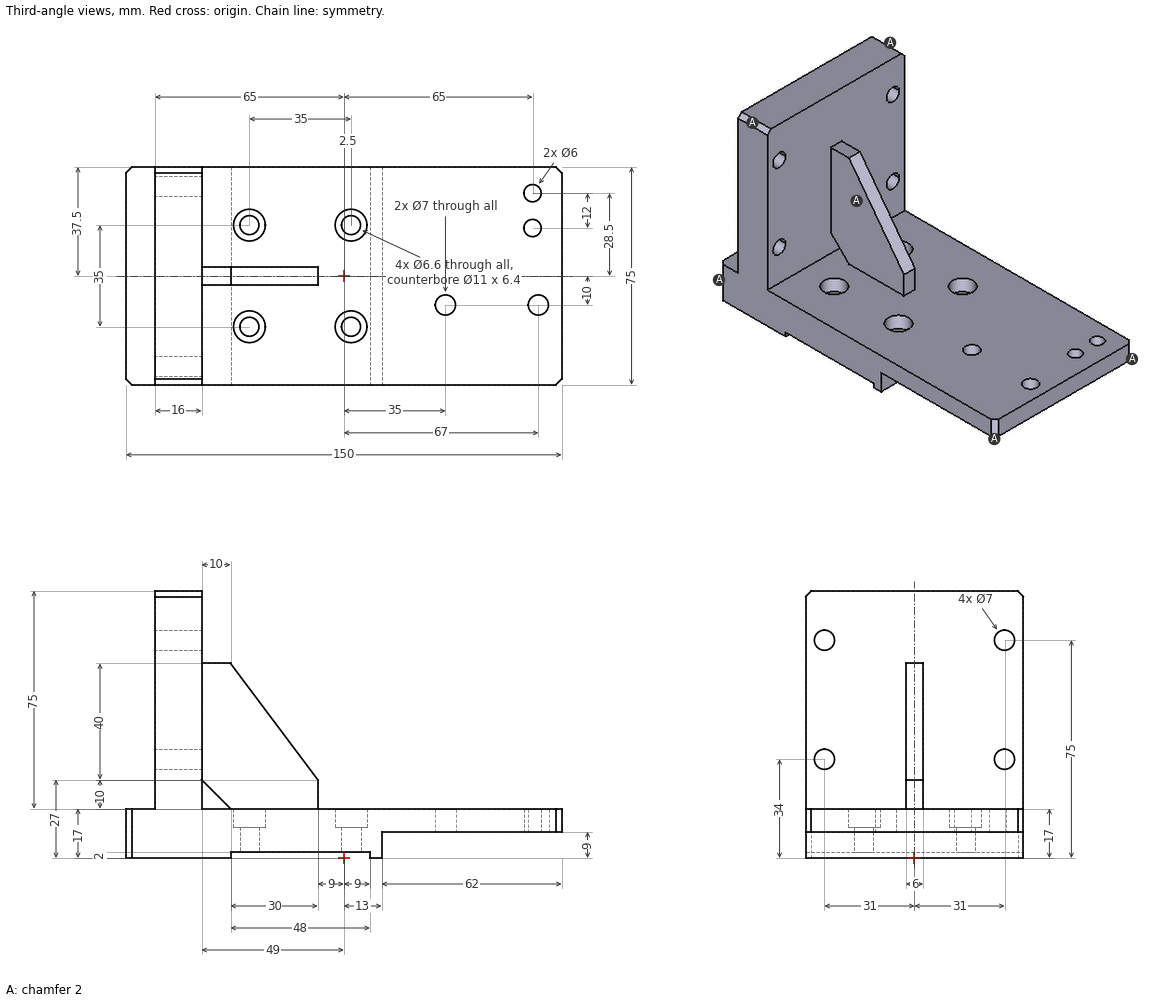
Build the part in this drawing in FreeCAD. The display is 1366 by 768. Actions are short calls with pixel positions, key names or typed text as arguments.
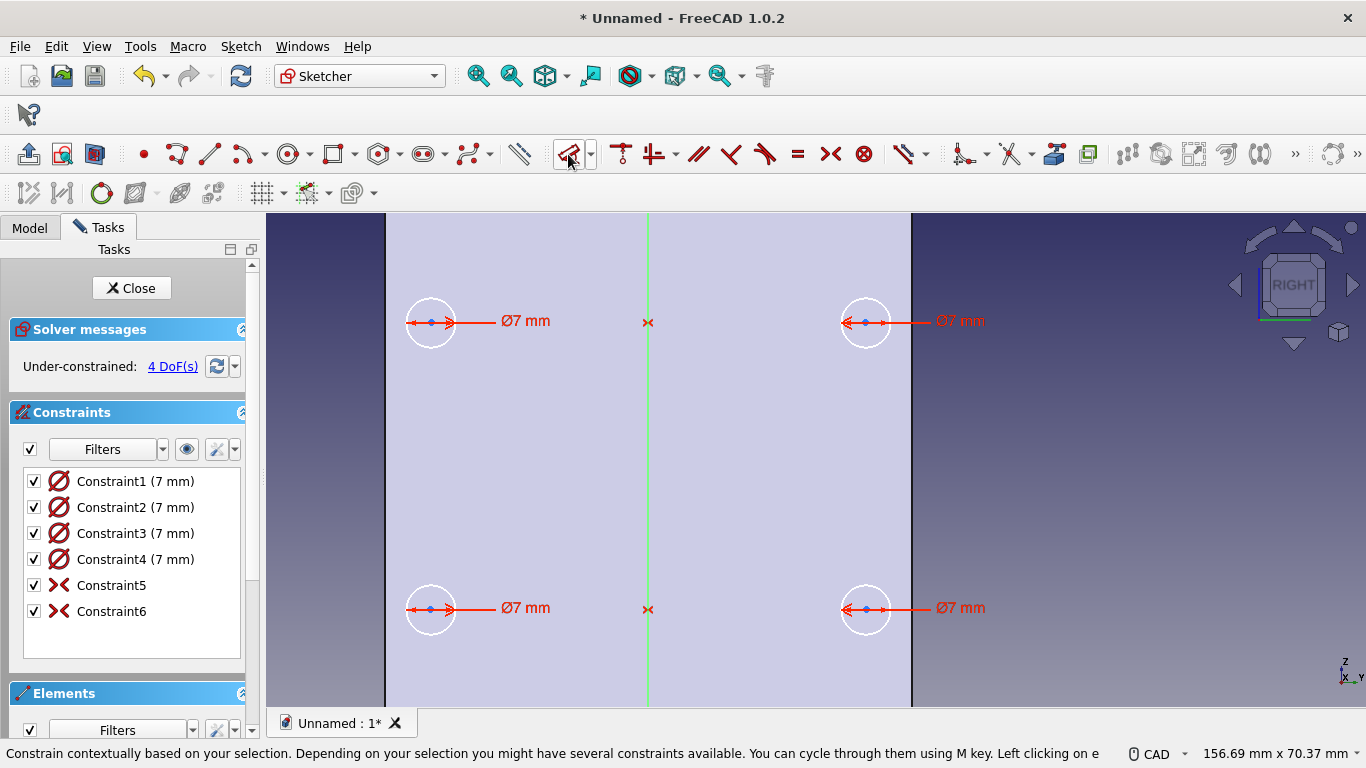
click(866, 323)
click(757, 289)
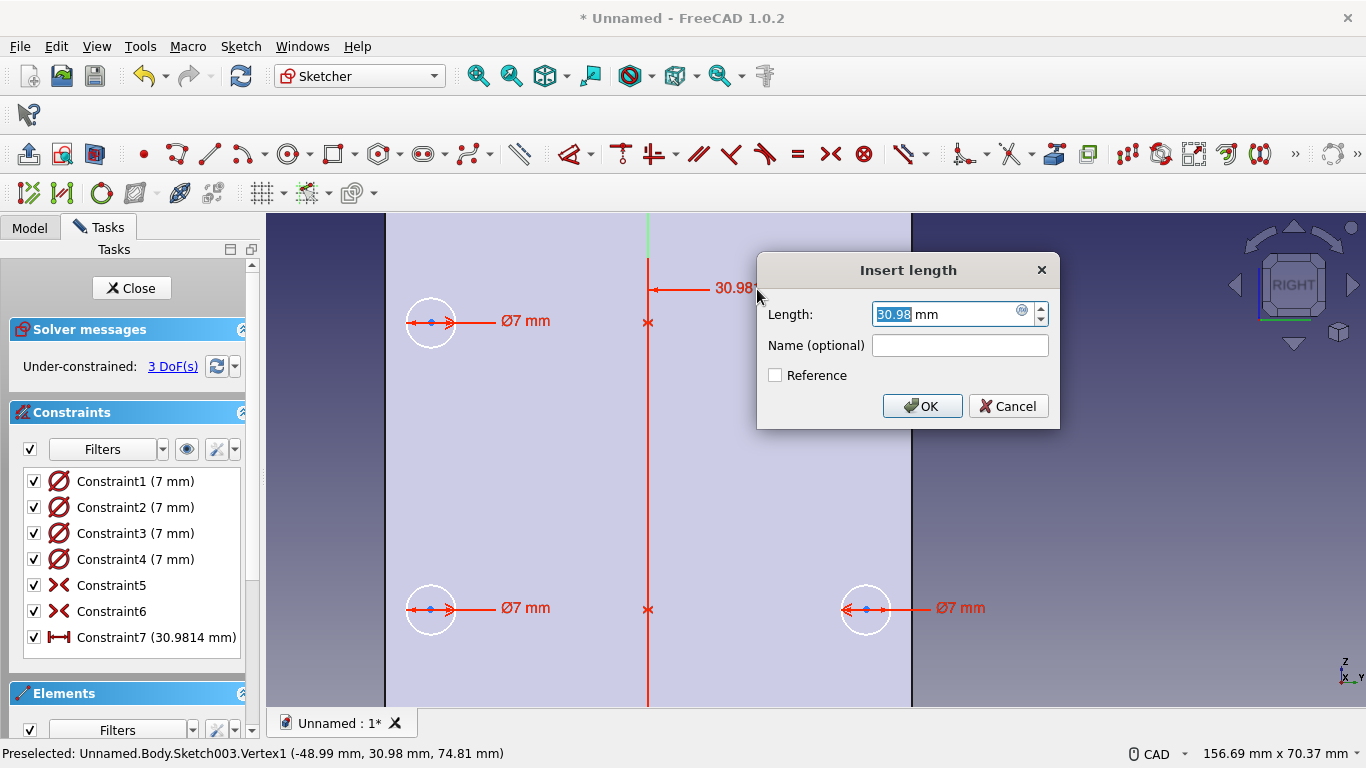
text(31)
key(Return)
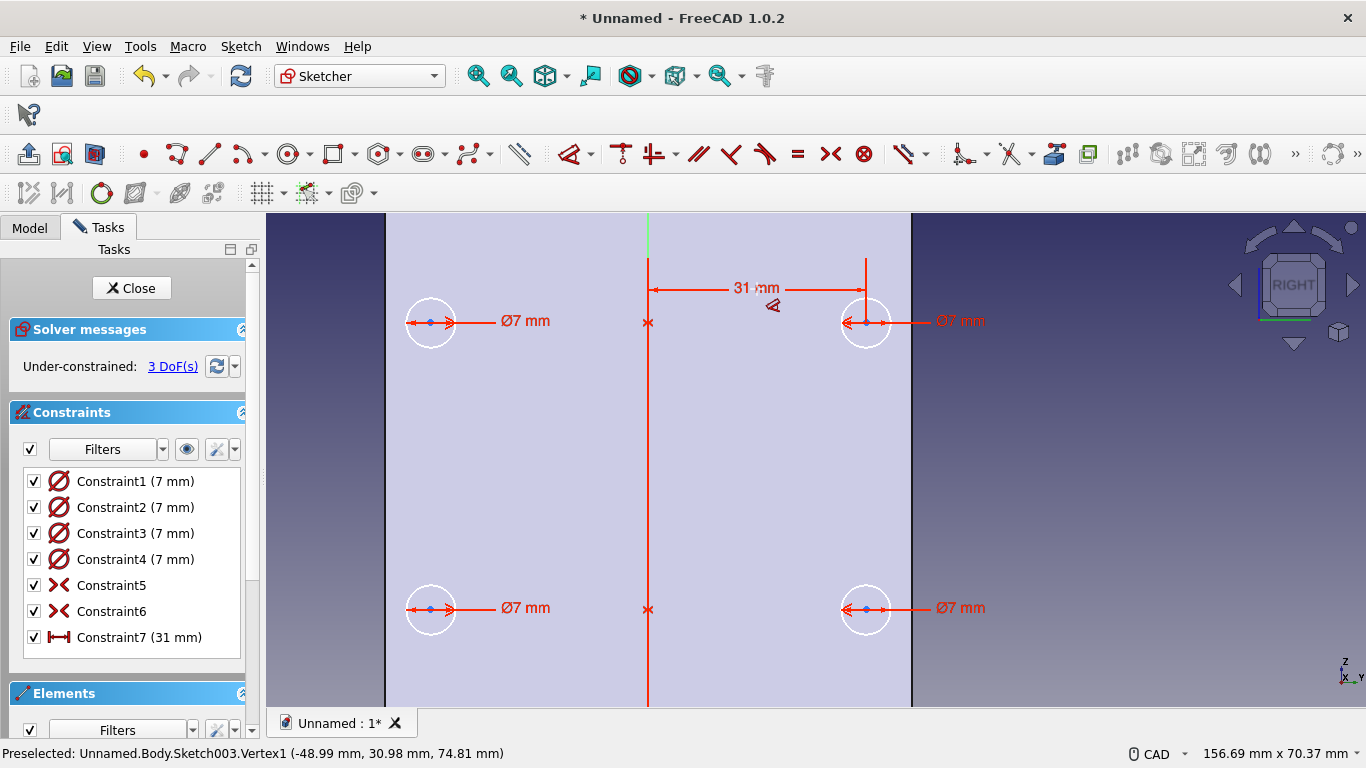
click(866, 323)
click(900, 501)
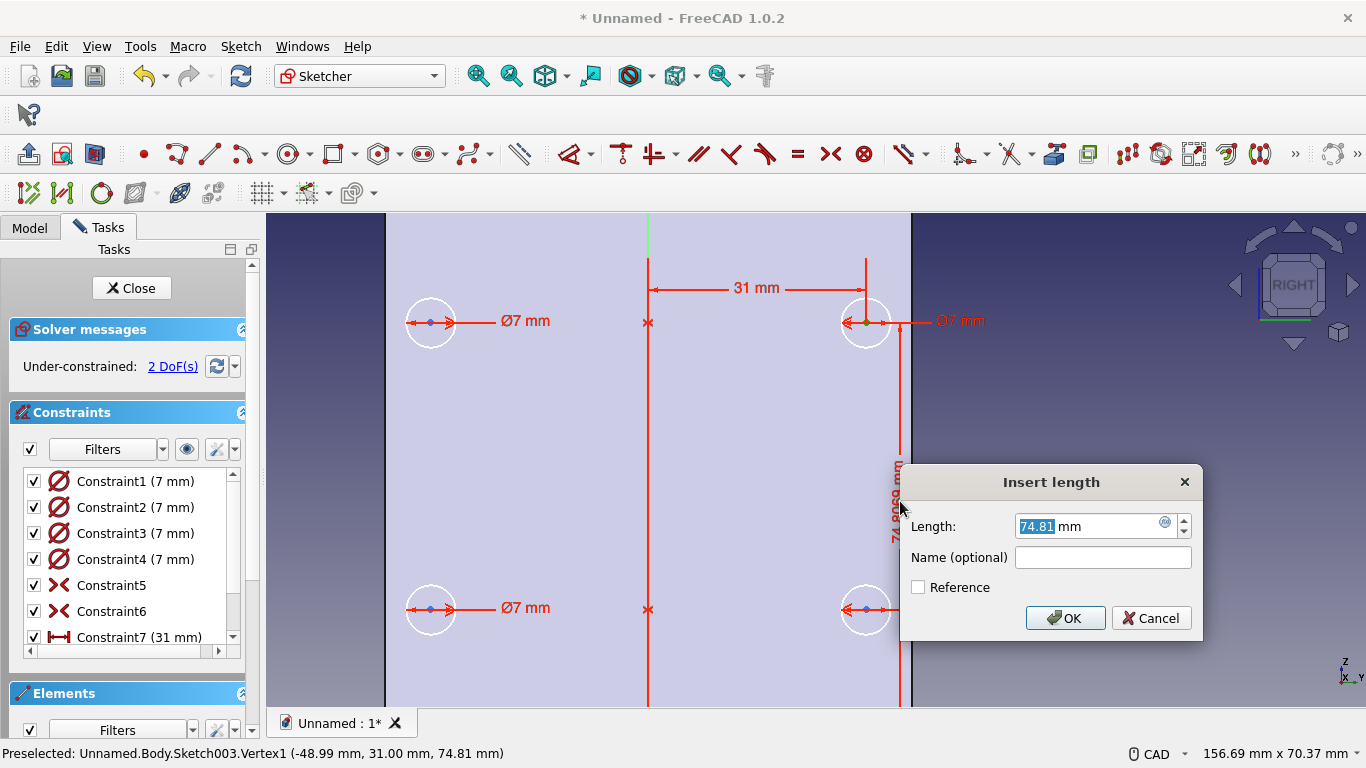
text(75)
key(Return)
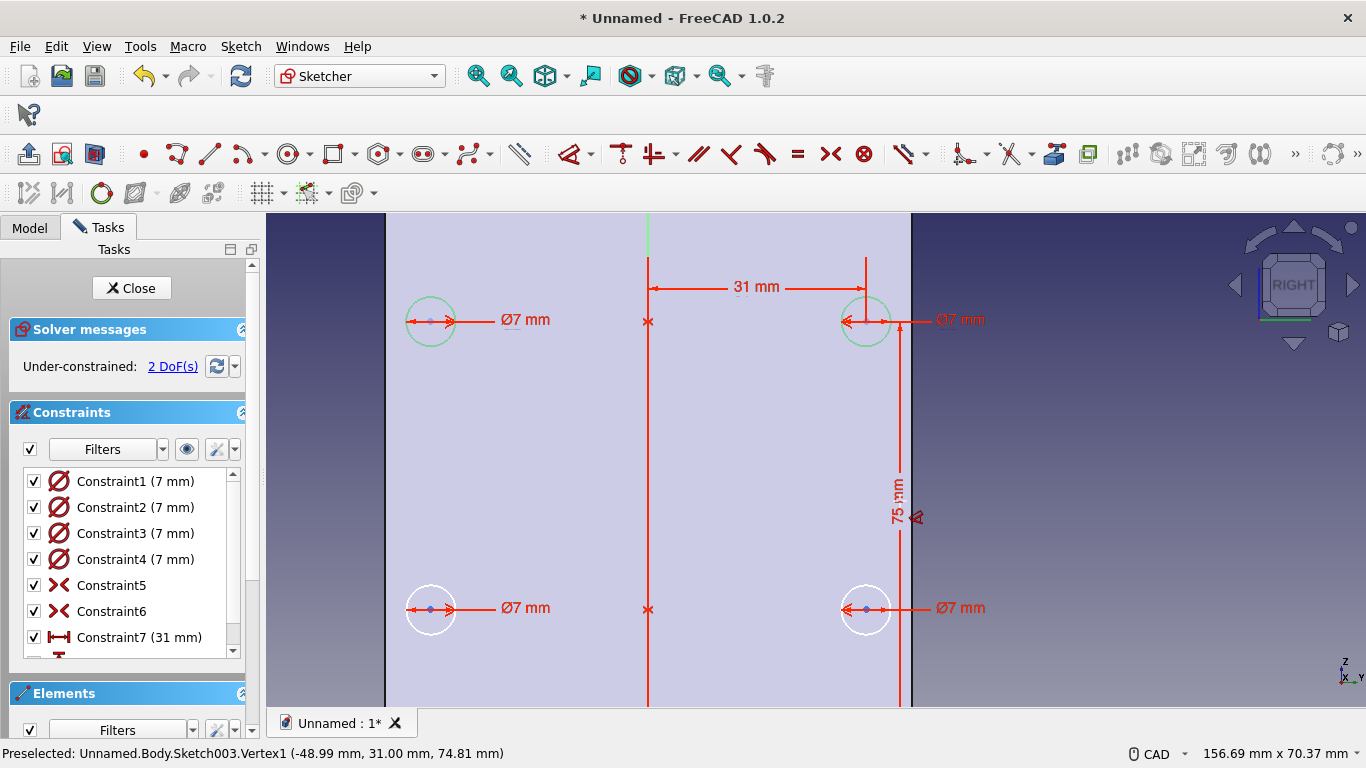
click(431, 610)
click(540, 576)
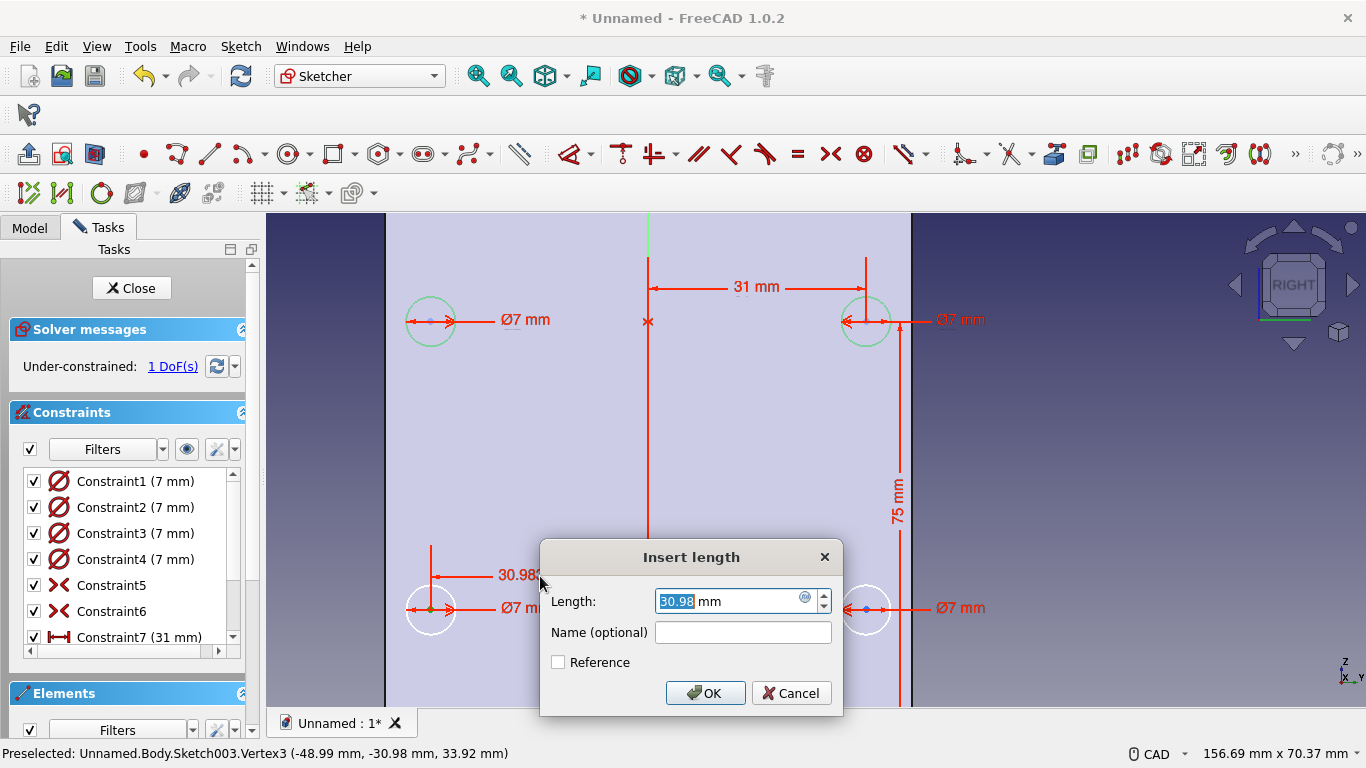
text(31)
key(Return)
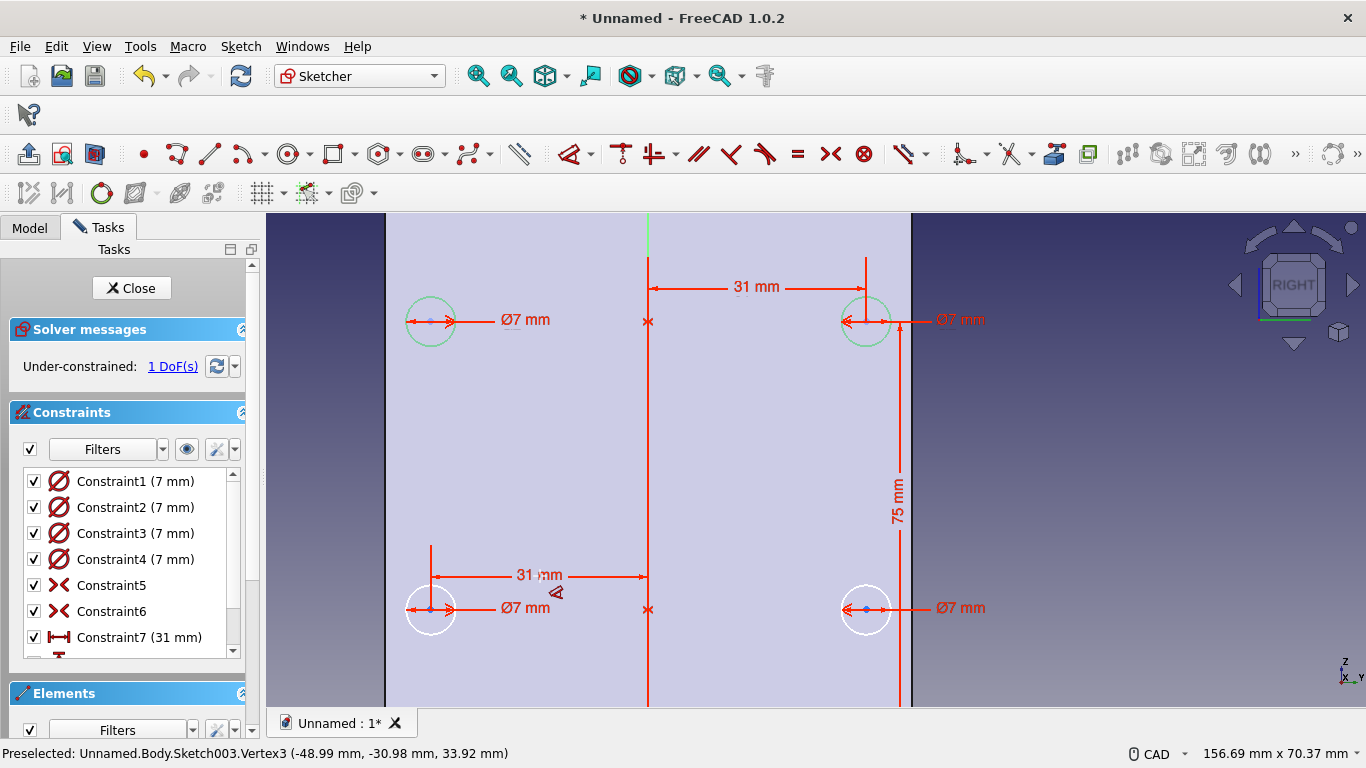
click(431, 610)
click(397, 644)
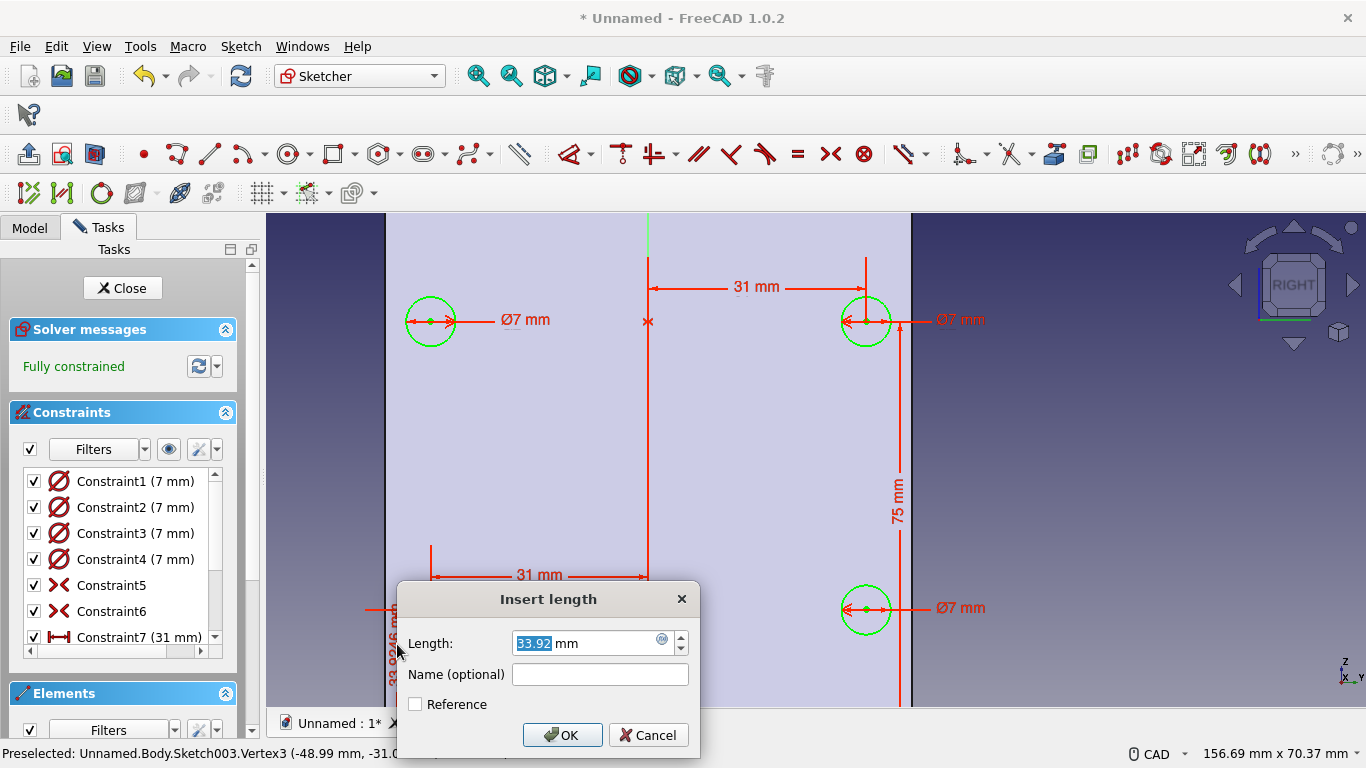
text(34)
key(Return)
key(Escape)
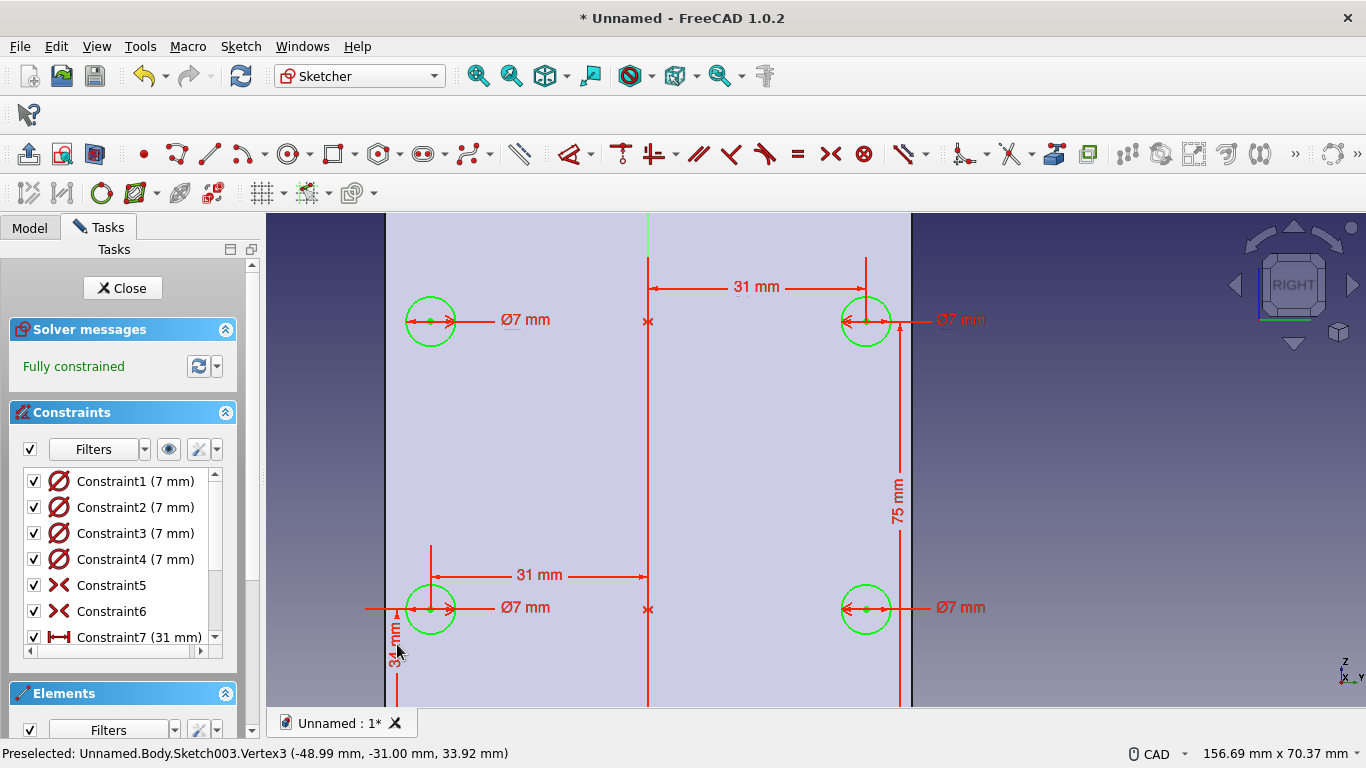
click(123, 288)